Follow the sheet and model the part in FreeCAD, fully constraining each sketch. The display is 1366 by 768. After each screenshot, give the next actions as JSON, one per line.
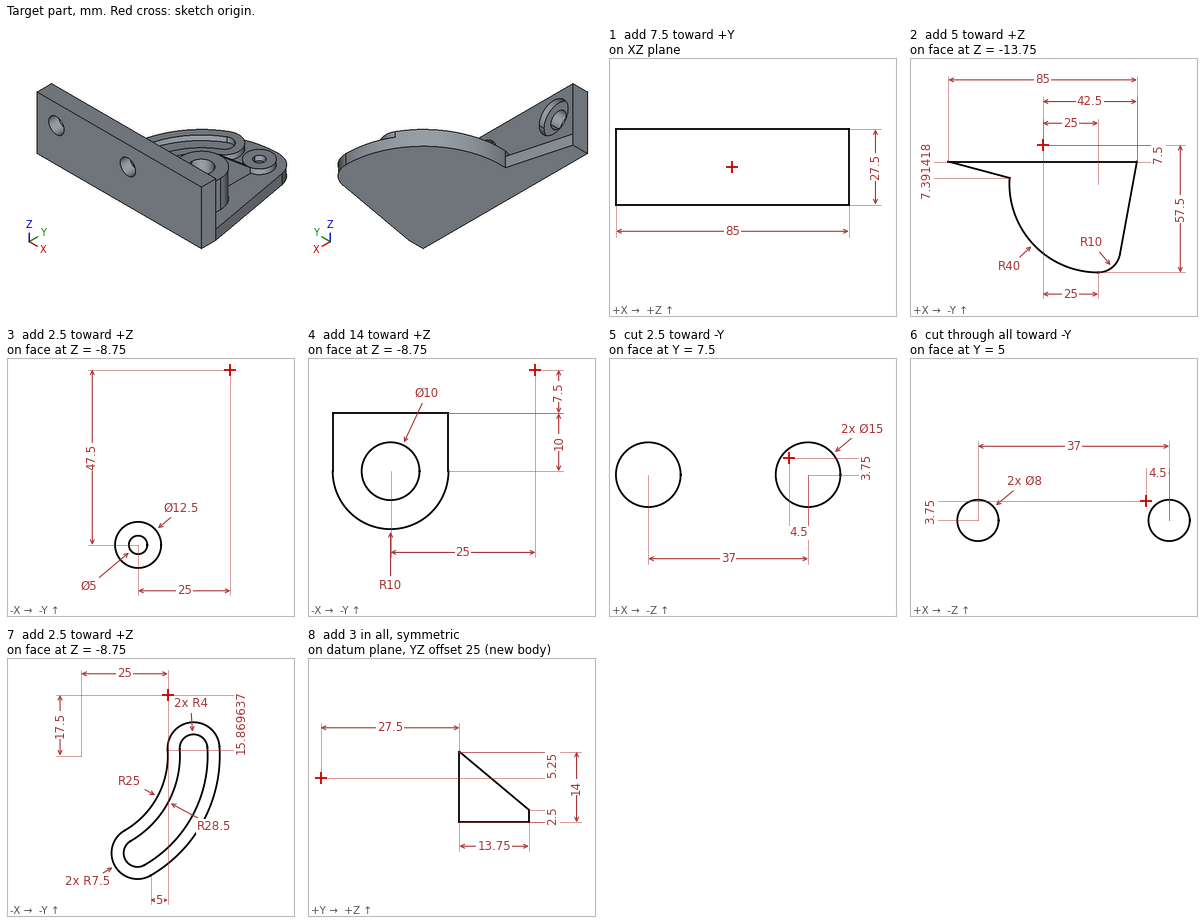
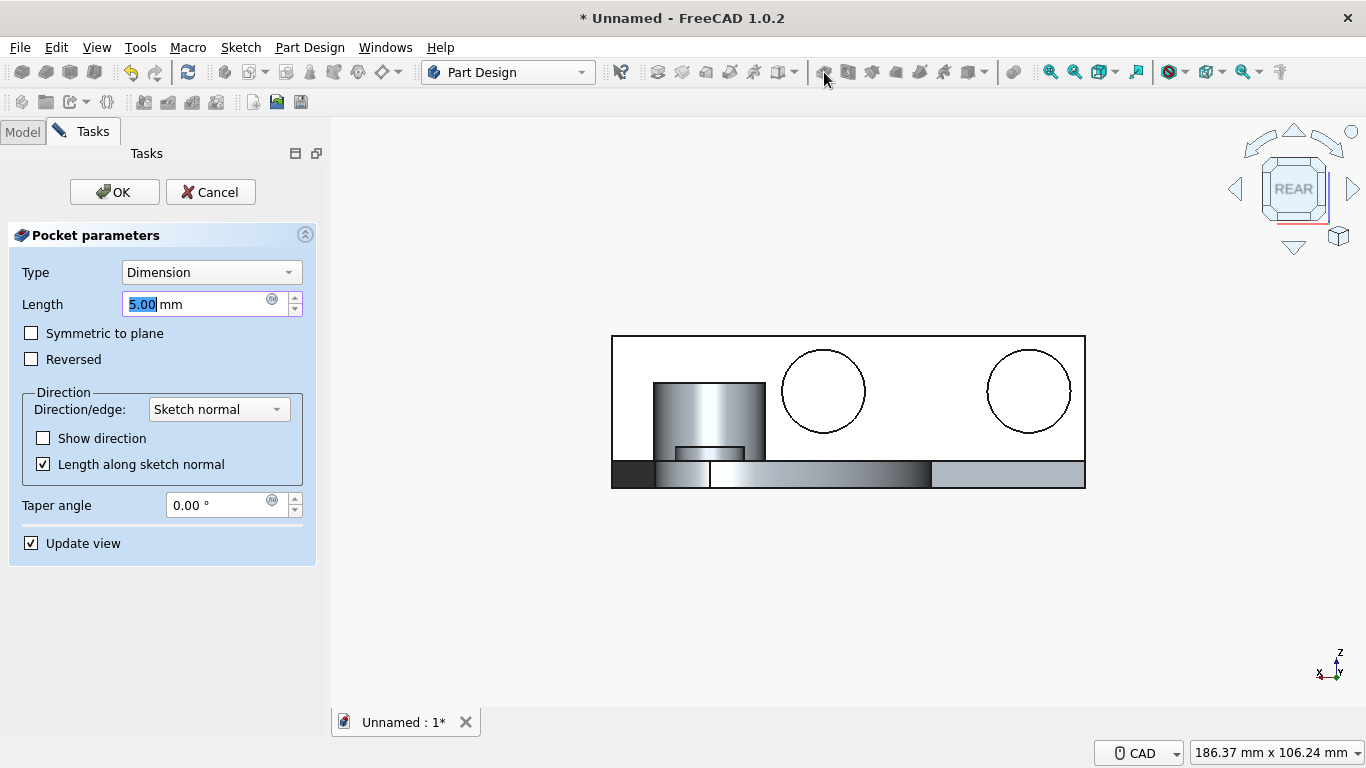
{"action": "type", "text": "2.5"}
{"action": "key", "text": "Tab"}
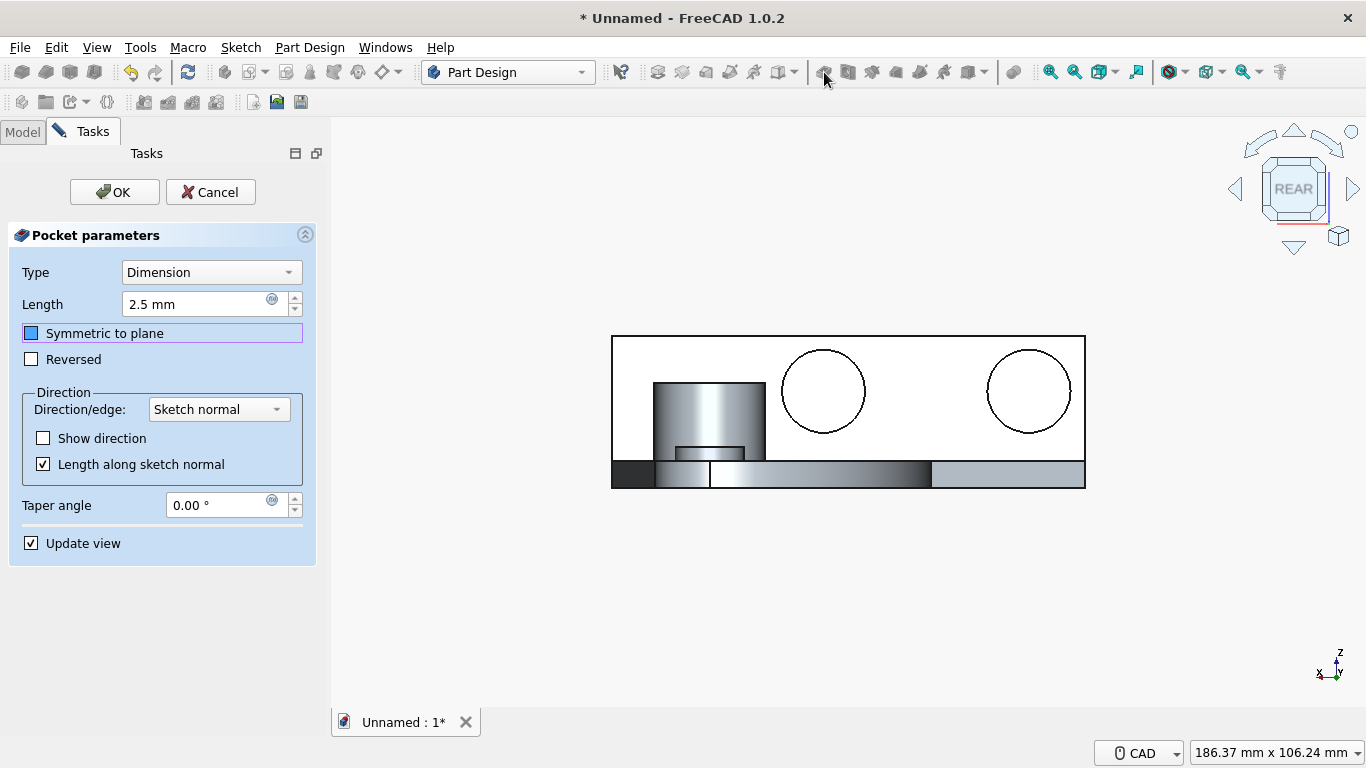
{"action": "left_click", "coordinate": [115, 192]}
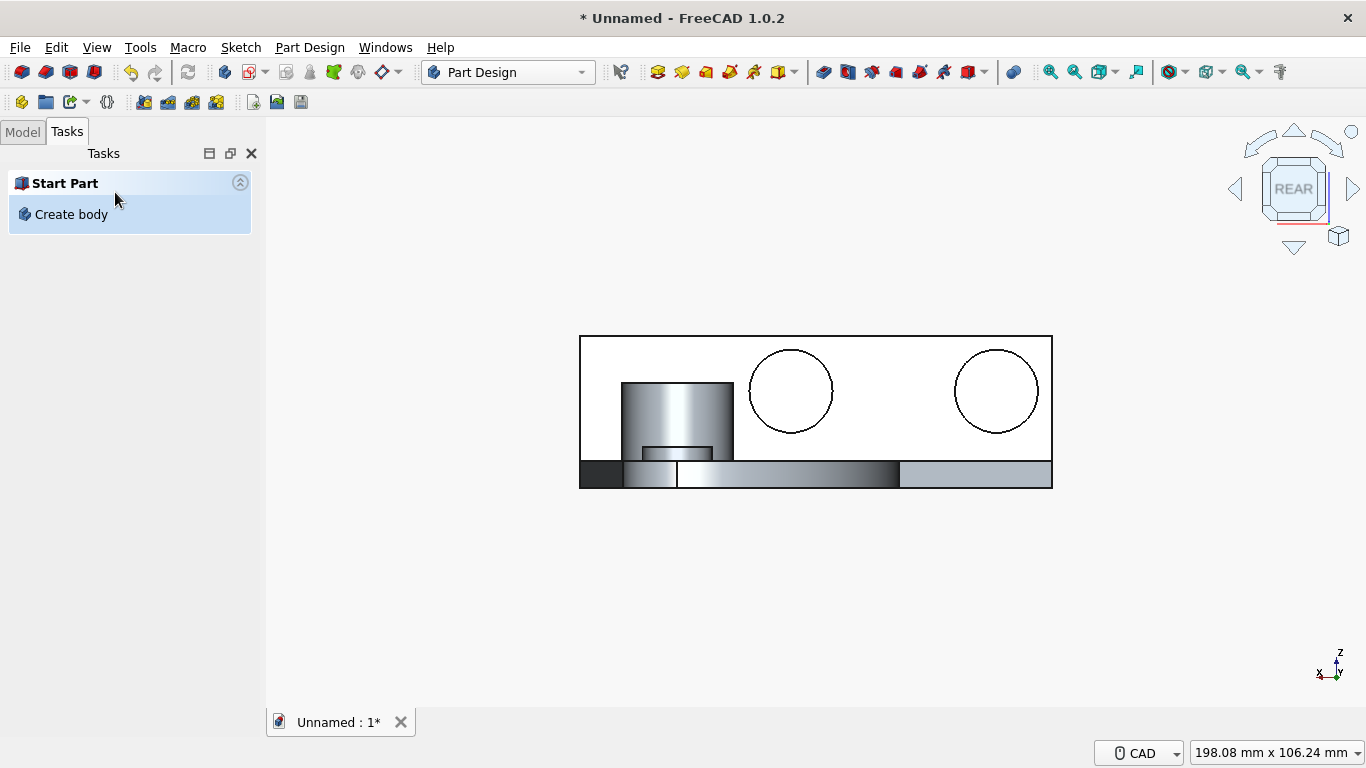
{"action": "left_click", "coordinate": [1052, 72]}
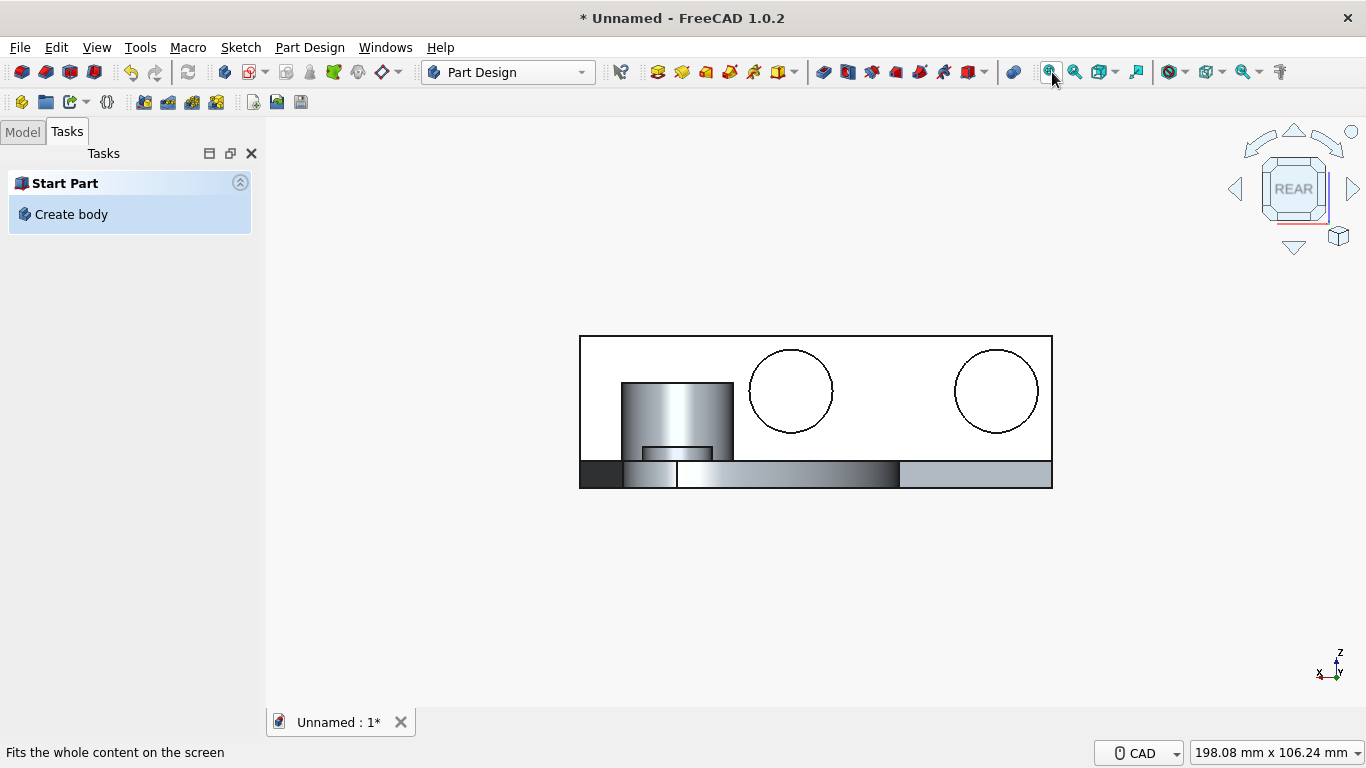
{"action": "left_click", "coordinate": [791, 390]}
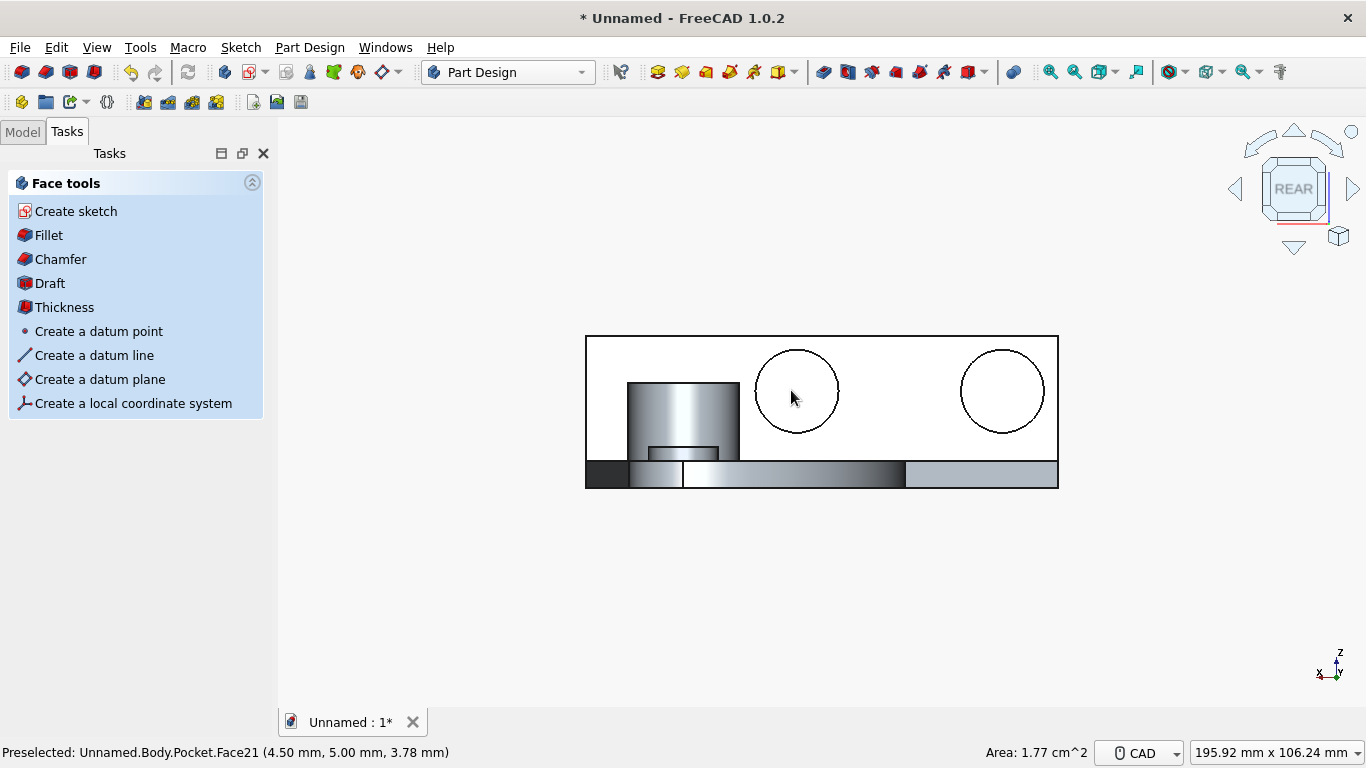
{"action": "left_click", "coordinate": [250, 72]}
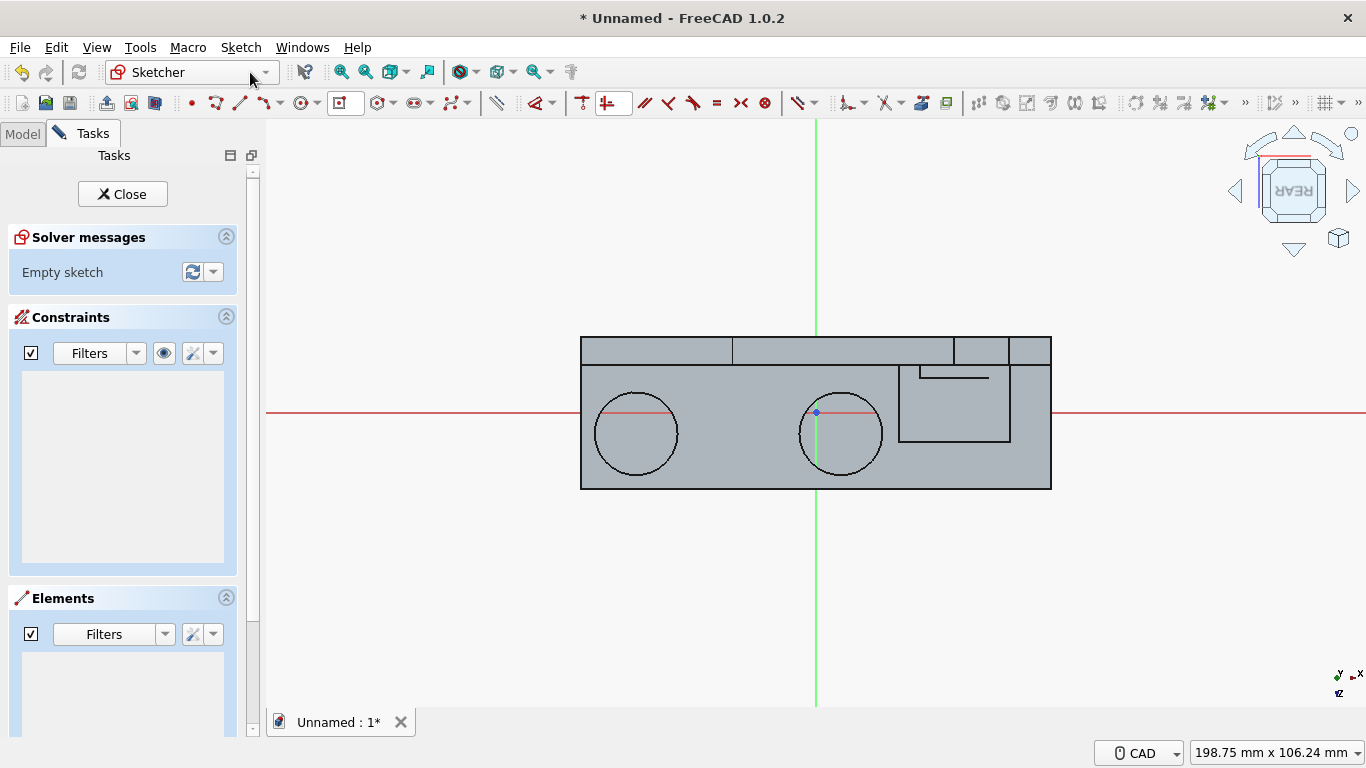
{"action": "scroll", "coordinate": [733, 446], "scroll_direction": "up", "scroll_amount": 5}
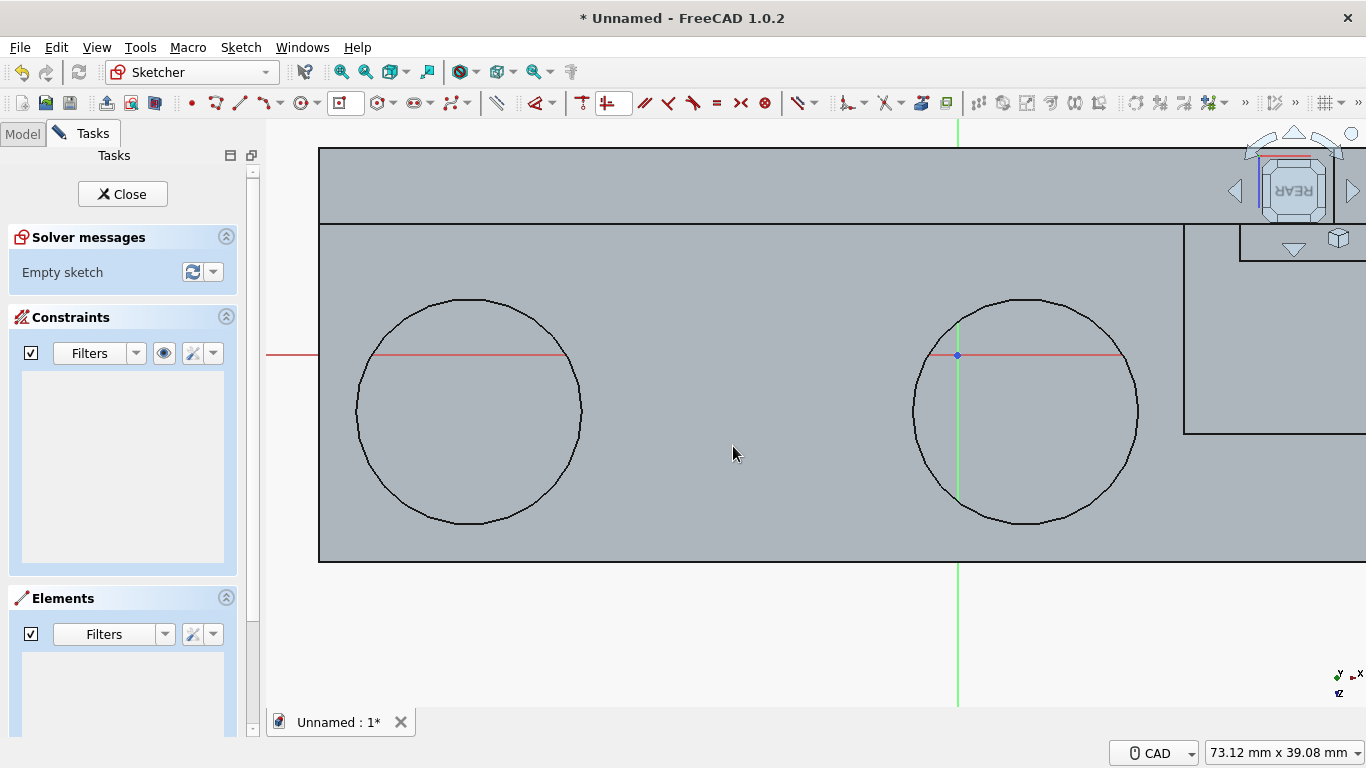
{"action": "left_click", "coordinate": [302, 104]}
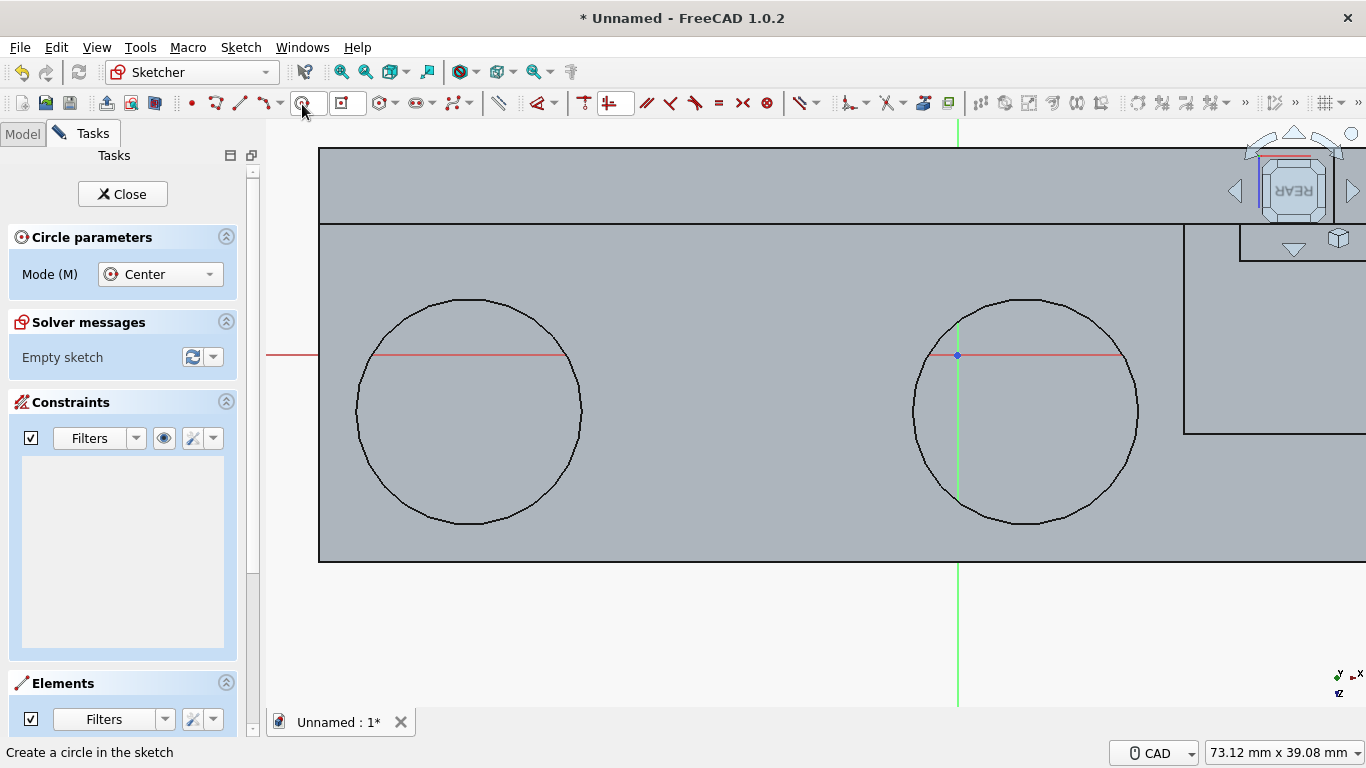
{"action": "left_click", "coordinate": [469, 412]}
{"action": "mouse_move", "coordinate": [511, 454]}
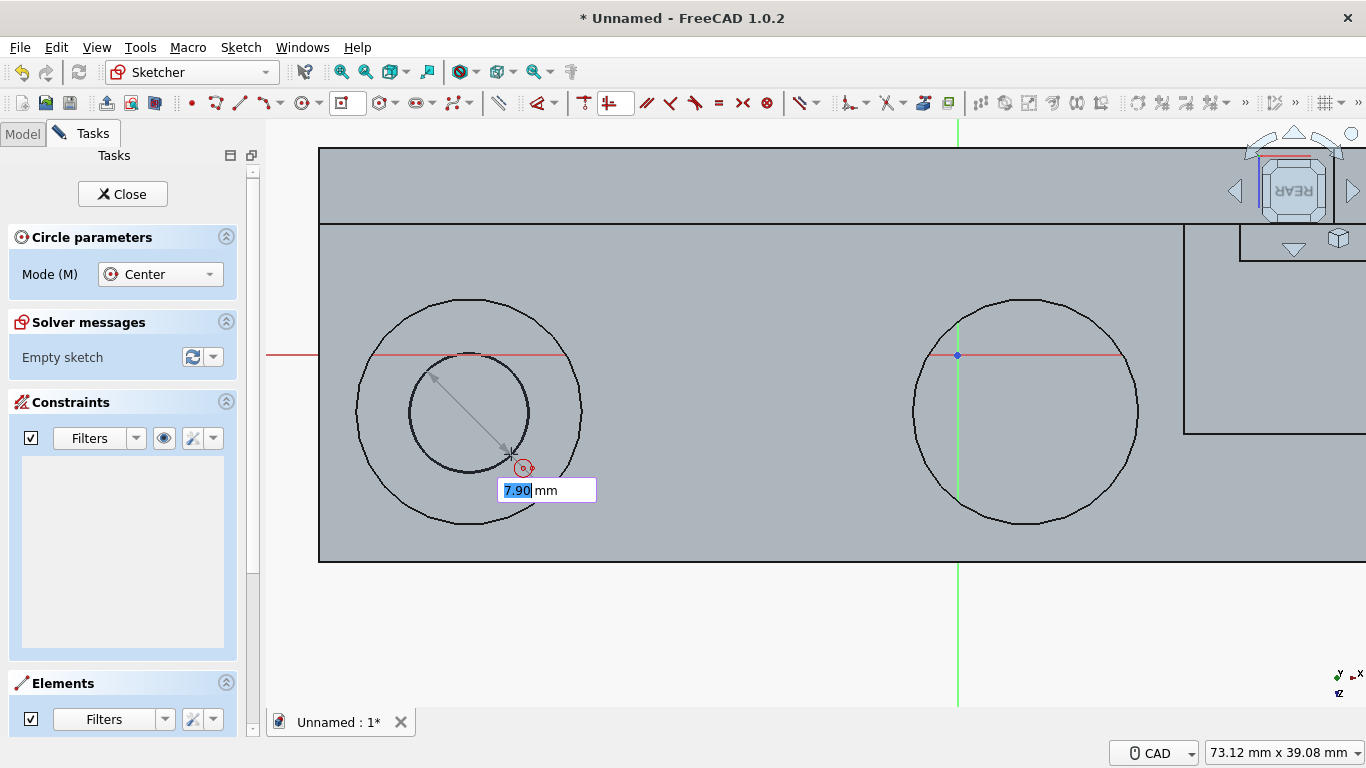
{"action": "type", "text": "8"}
{"action": "key", "text": "Return"}